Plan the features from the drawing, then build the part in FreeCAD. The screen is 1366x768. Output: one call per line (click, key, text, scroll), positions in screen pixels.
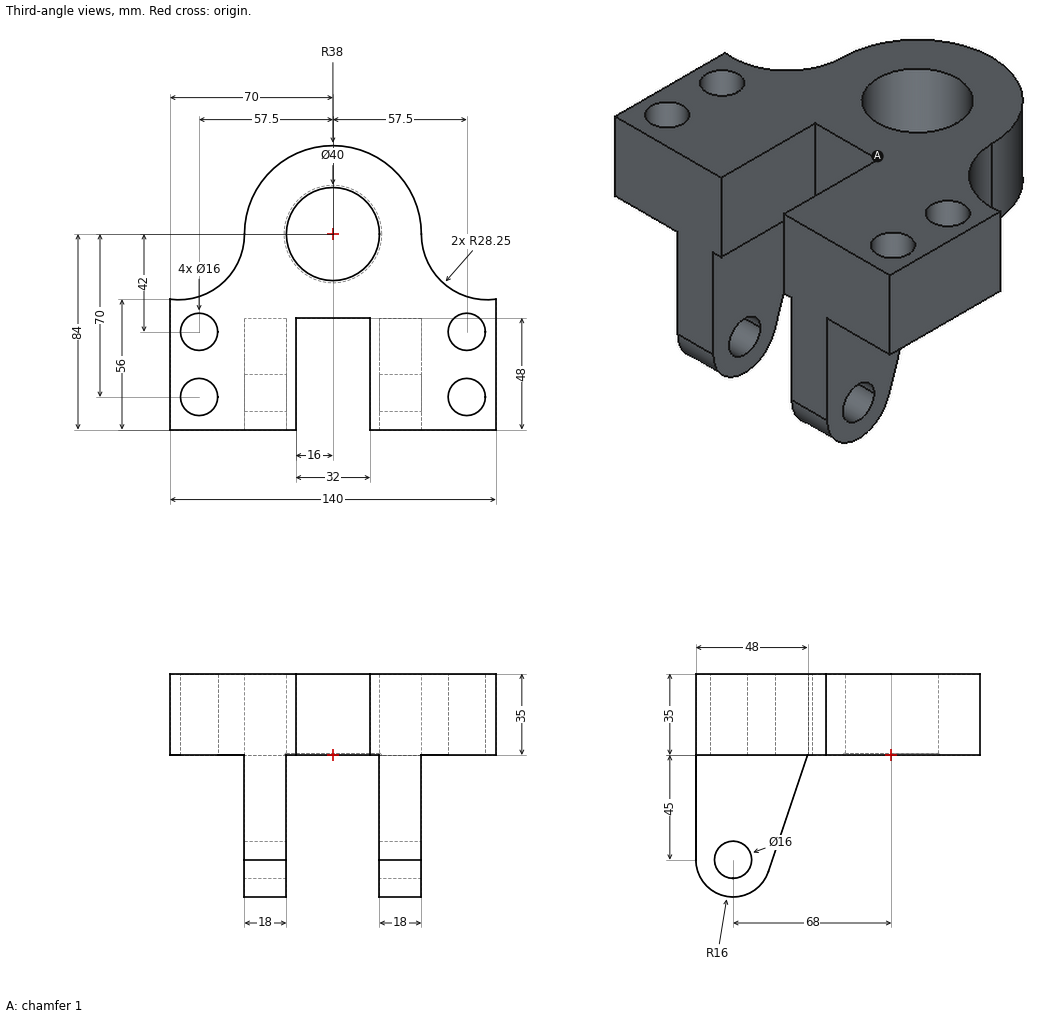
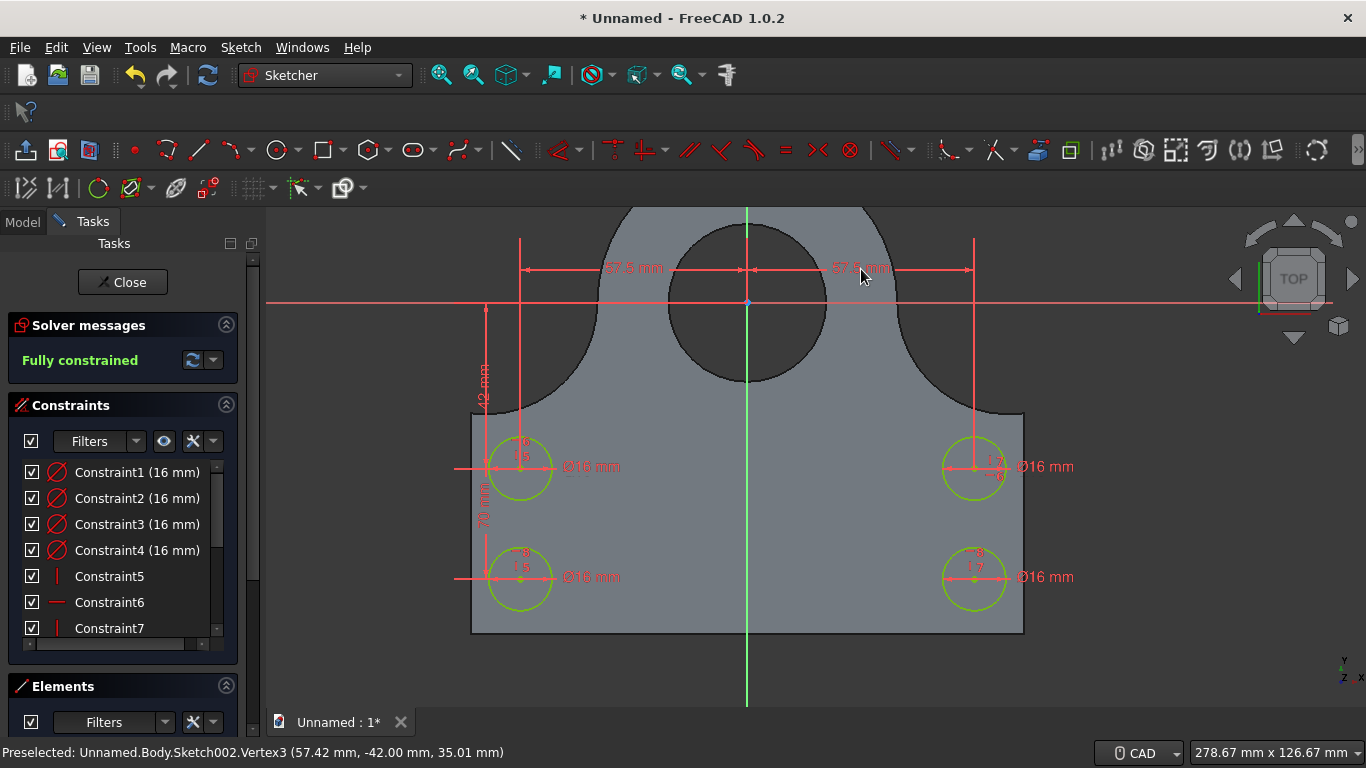
click(123, 282)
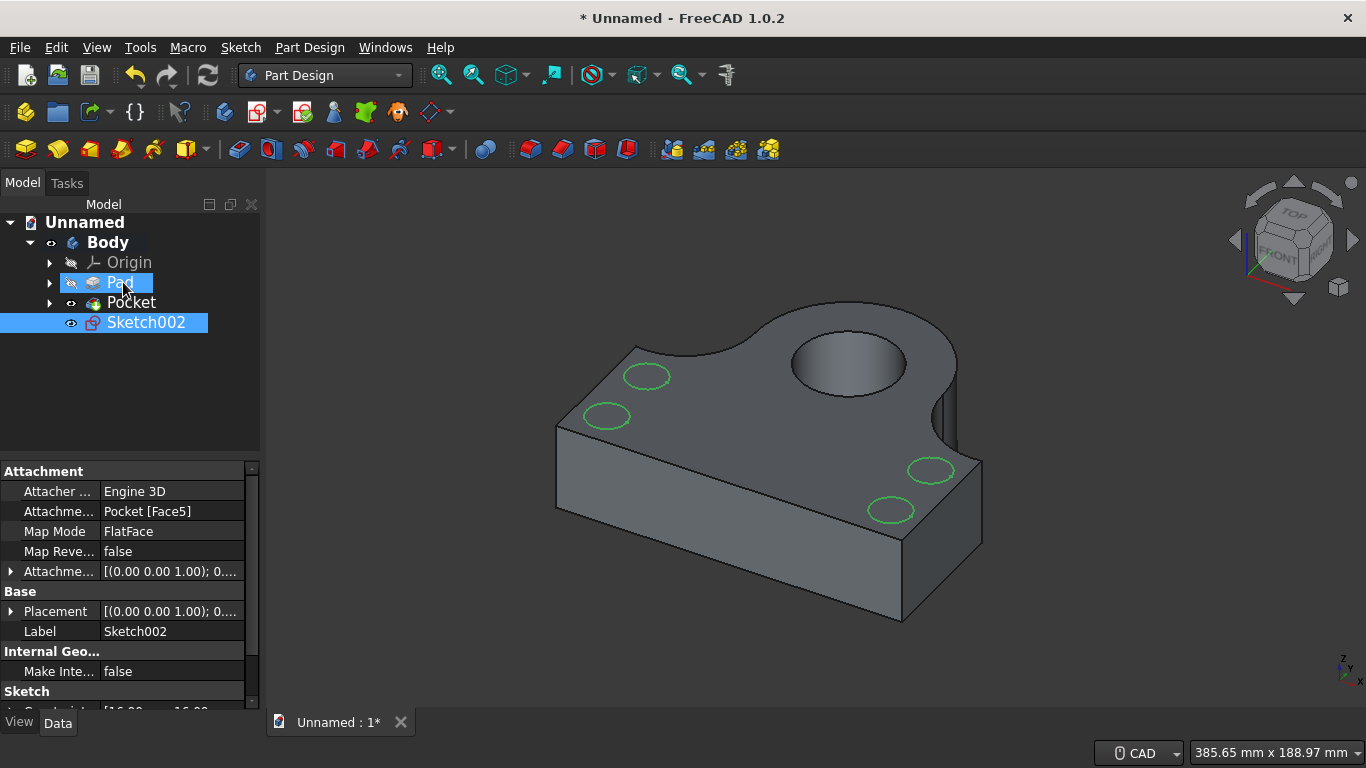
click(240, 150)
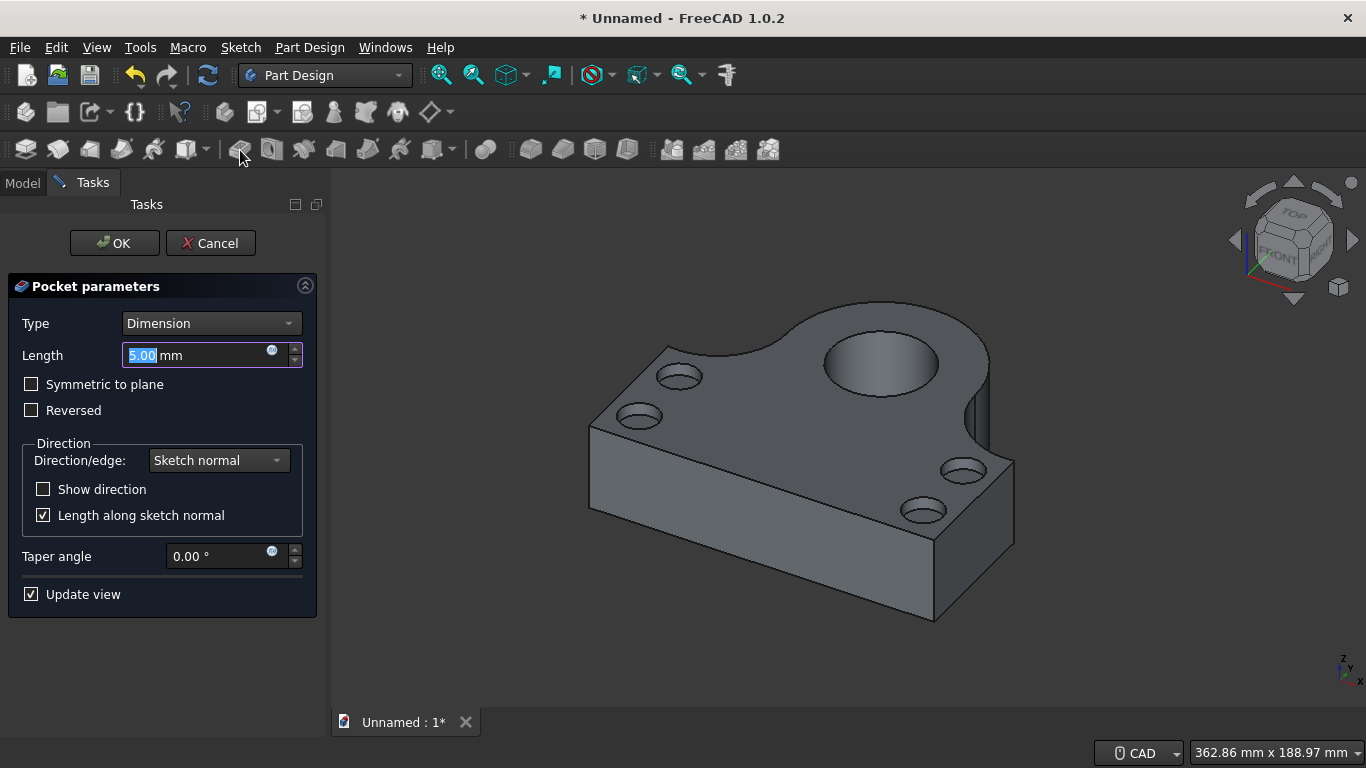
text(35)
key(Tab)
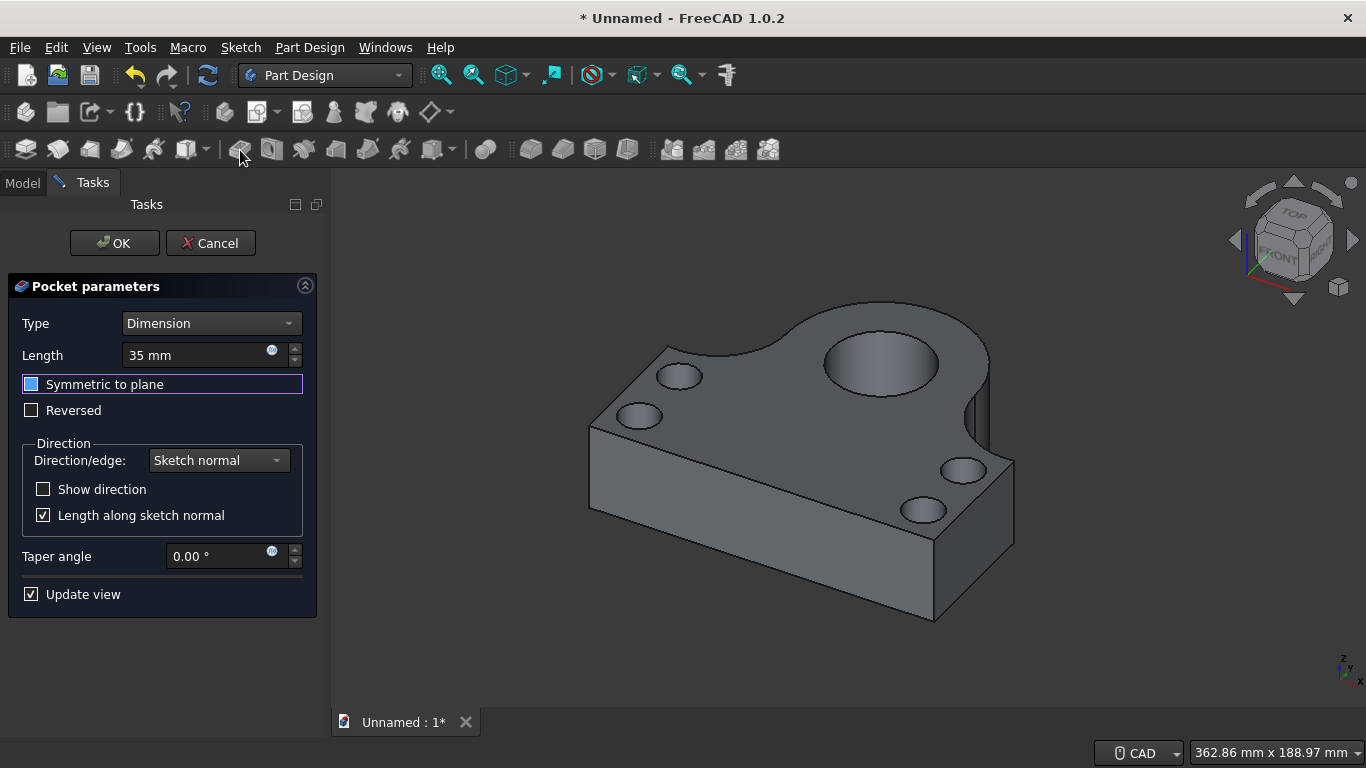
click(115, 243)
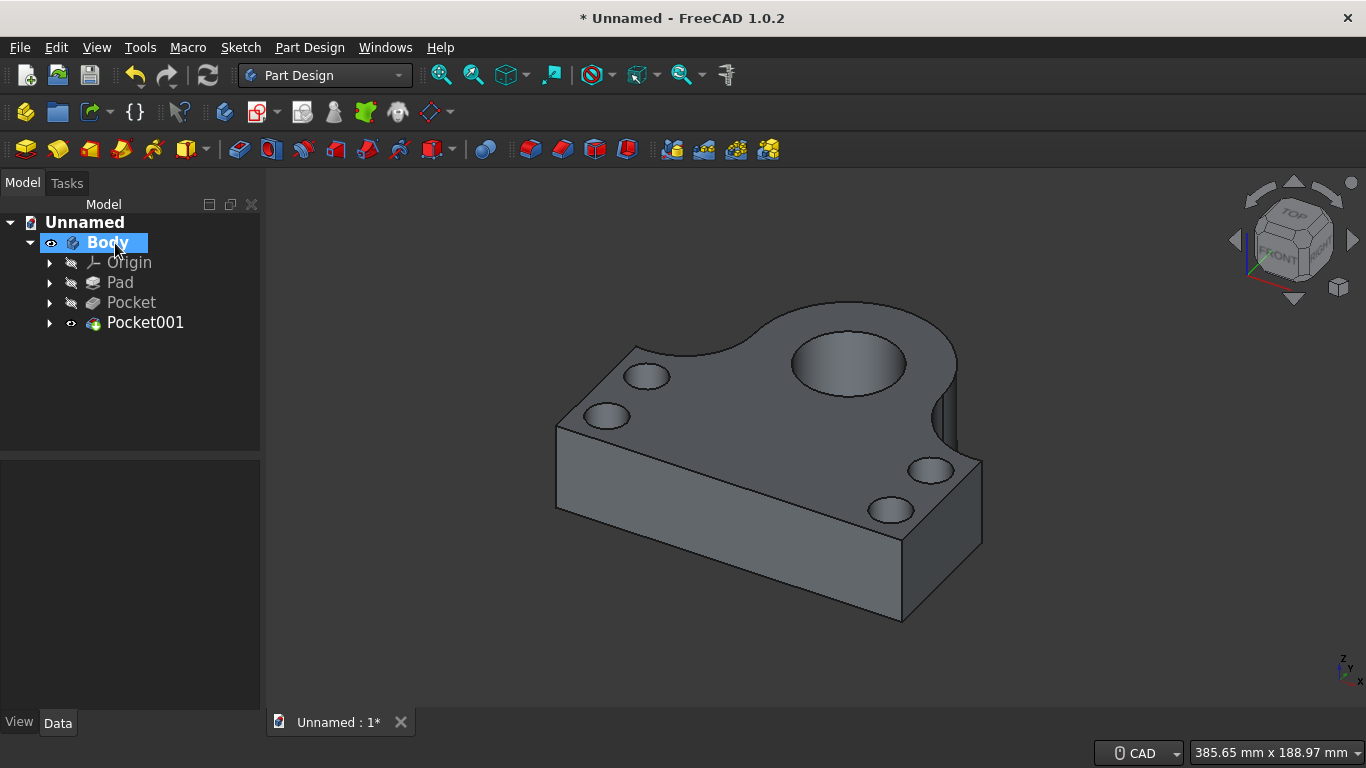
click(50, 263)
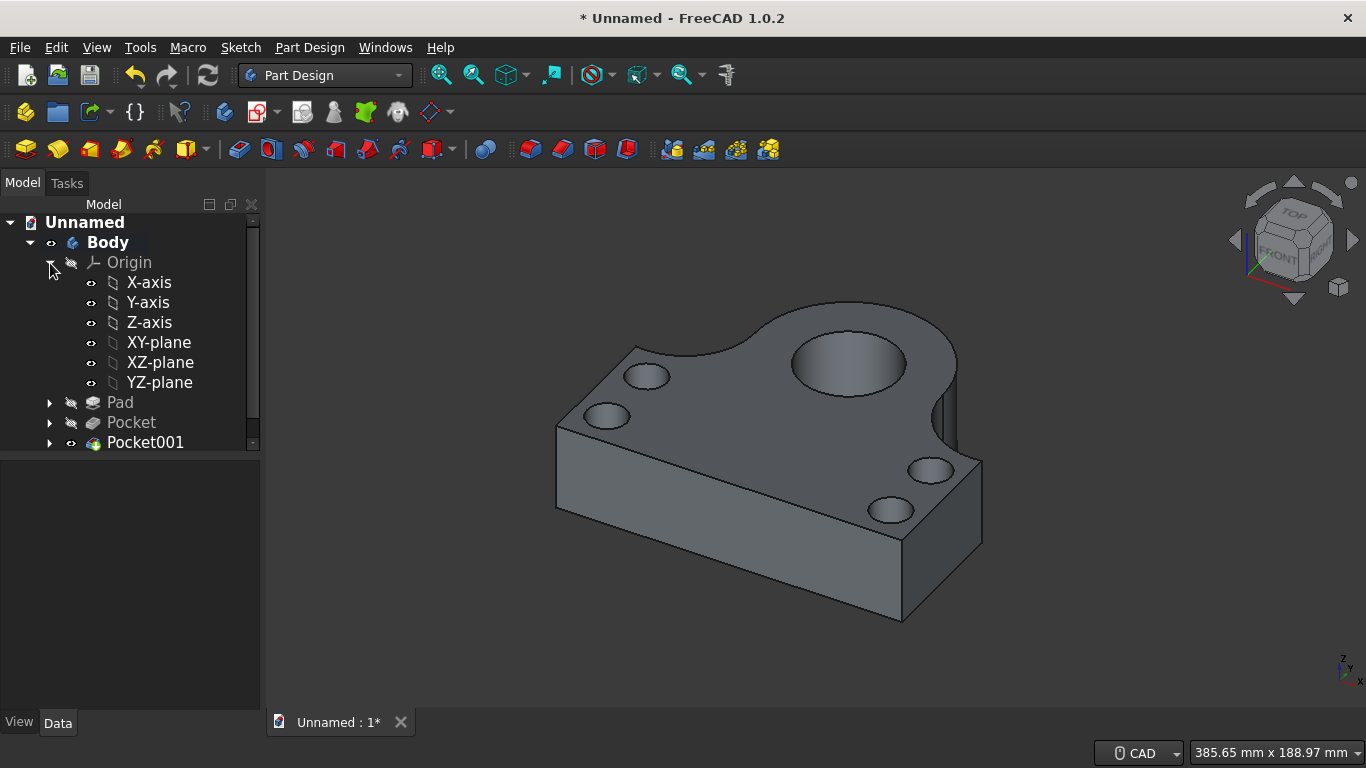
click(136, 383)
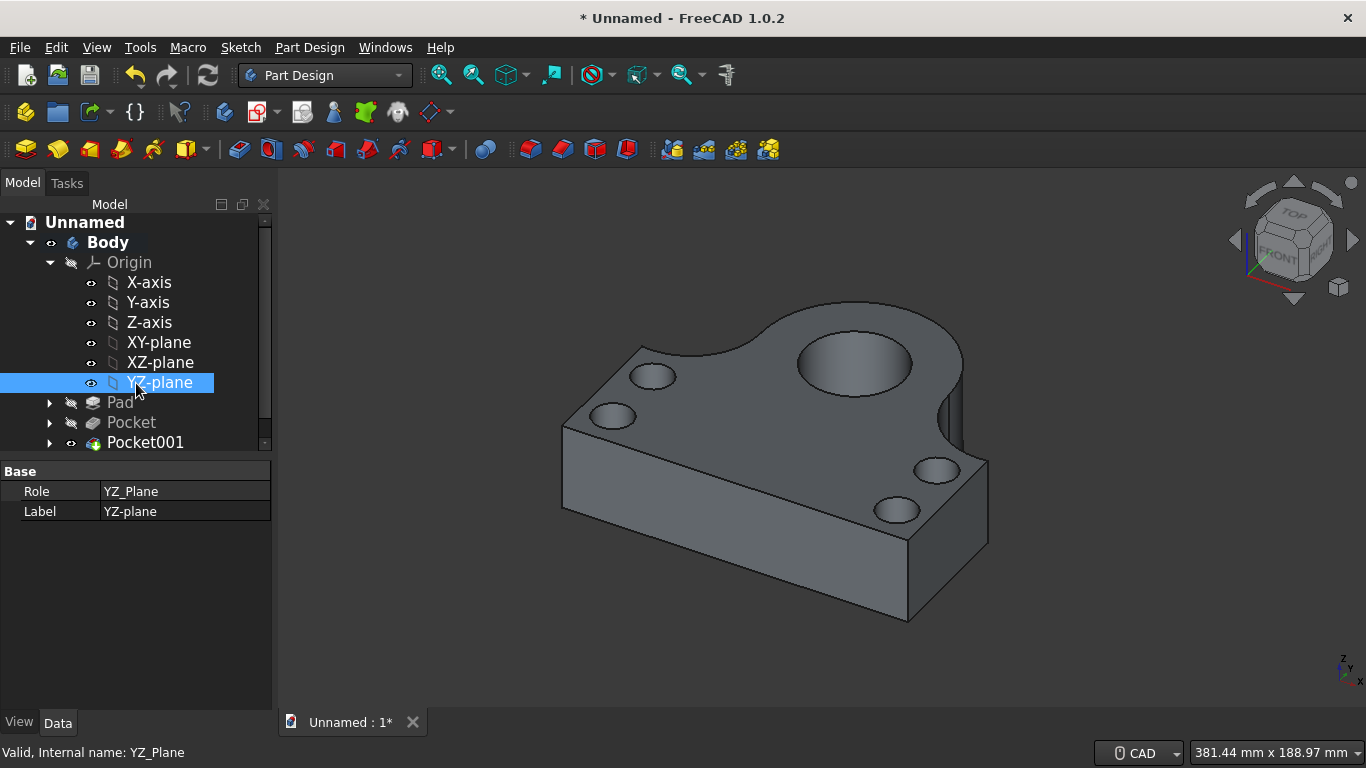
click(430, 112)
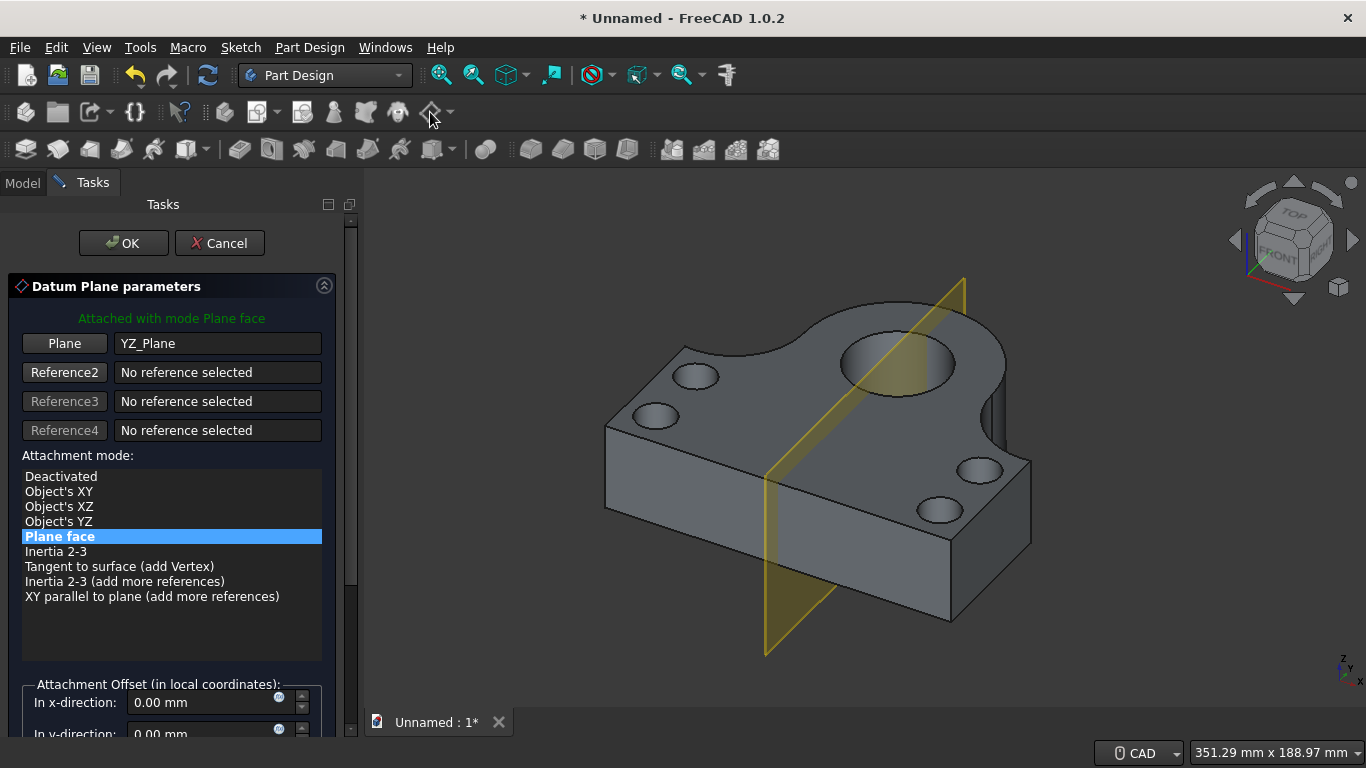
scroll(351, 475, down, 2)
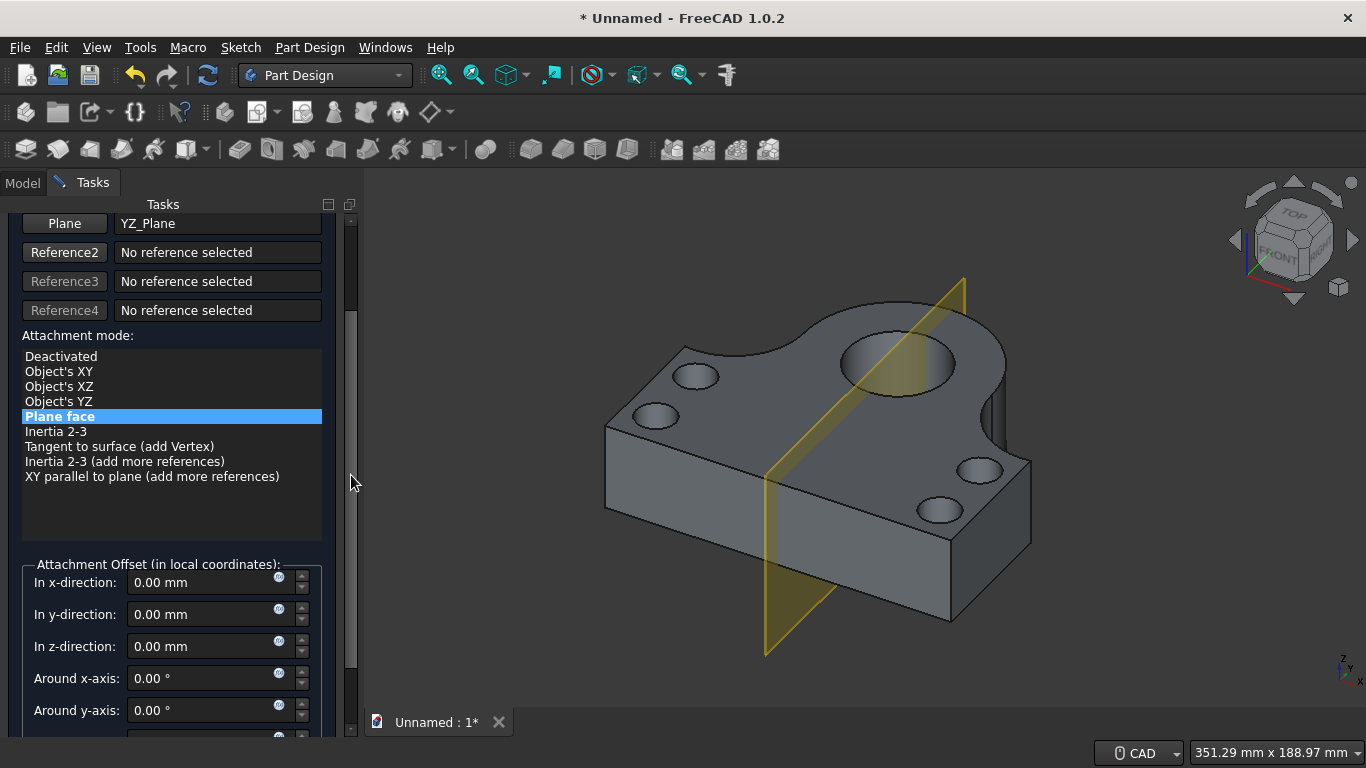
triple_click(210, 646)